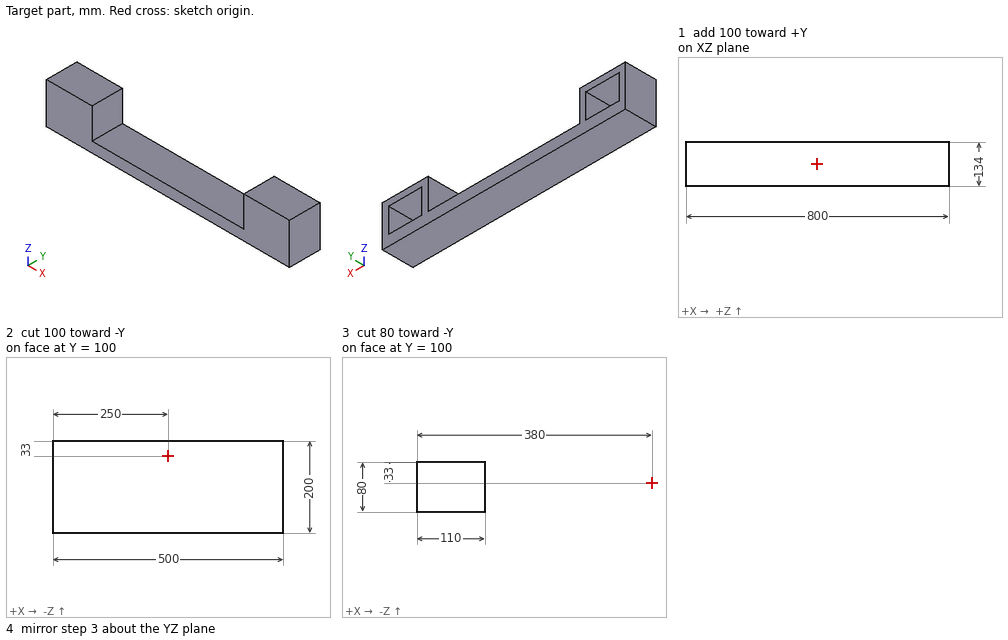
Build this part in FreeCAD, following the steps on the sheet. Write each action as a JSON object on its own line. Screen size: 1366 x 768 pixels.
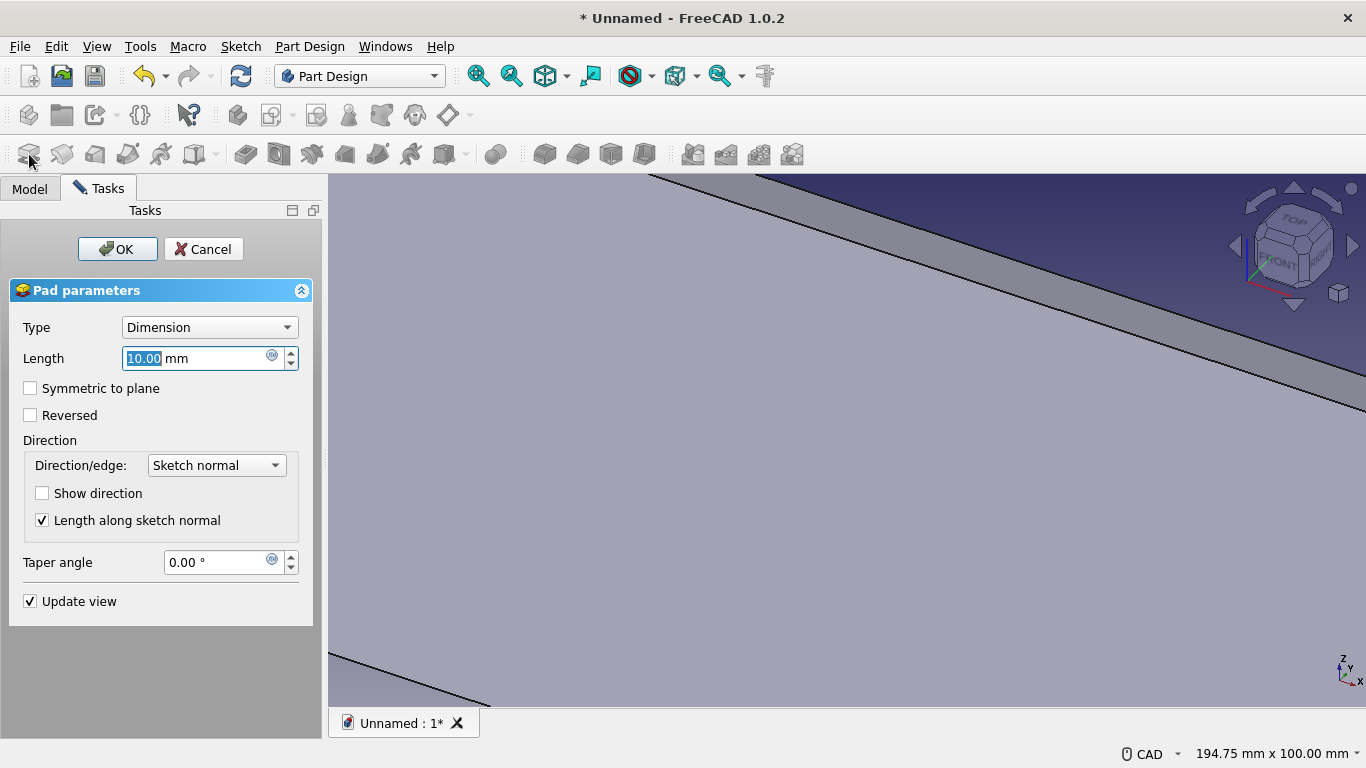
{"action": "type", "text": "100"}
{"action": "key", "text": "Tab"}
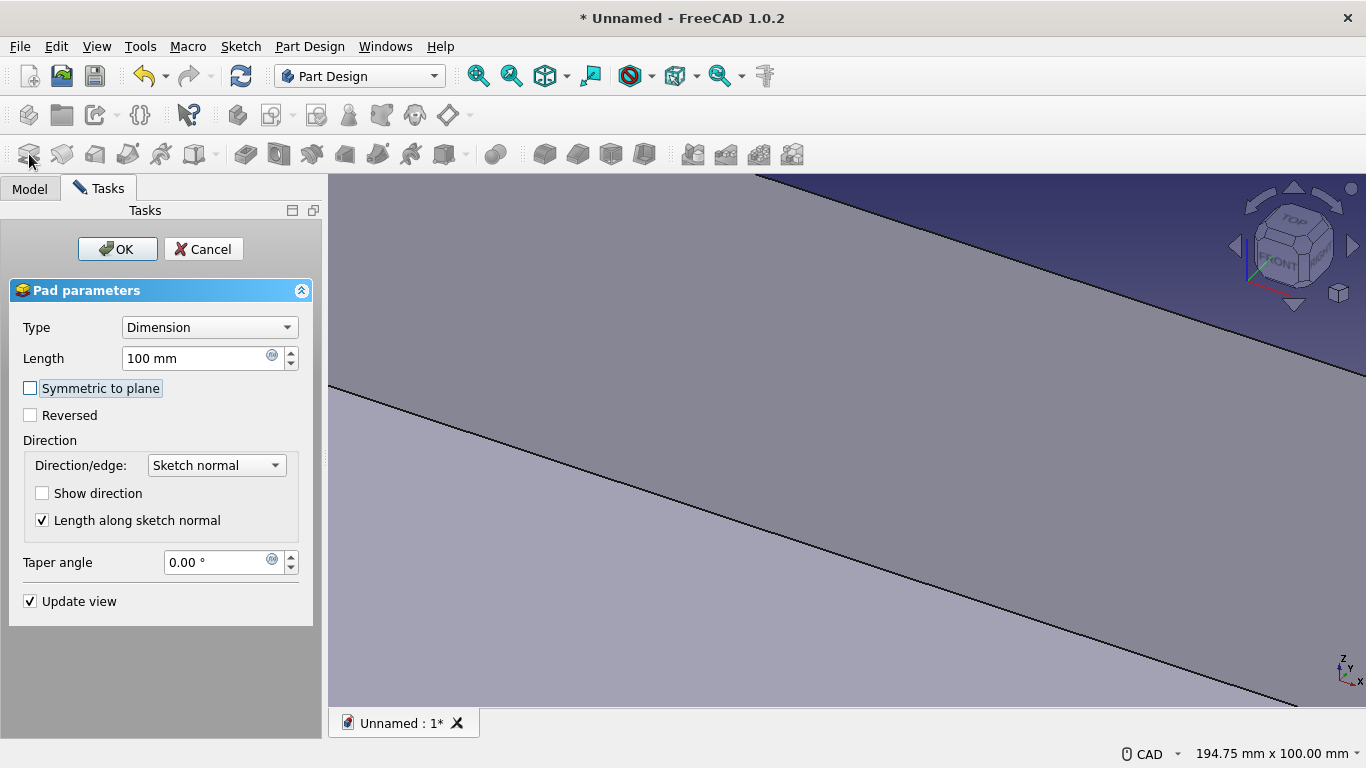
{"action": "left_click", "coordinate": [31, 415]}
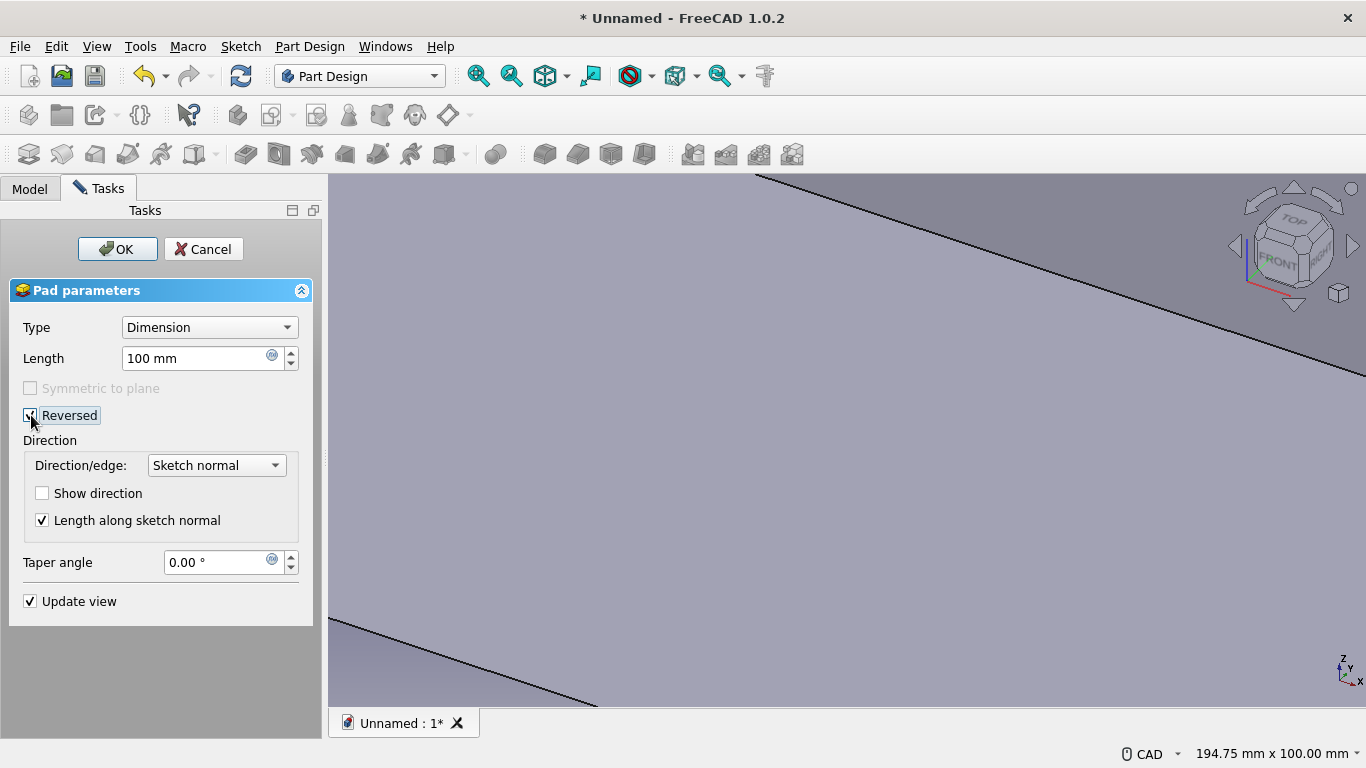
{"action": "left_click", "coordinate": [118, 249]}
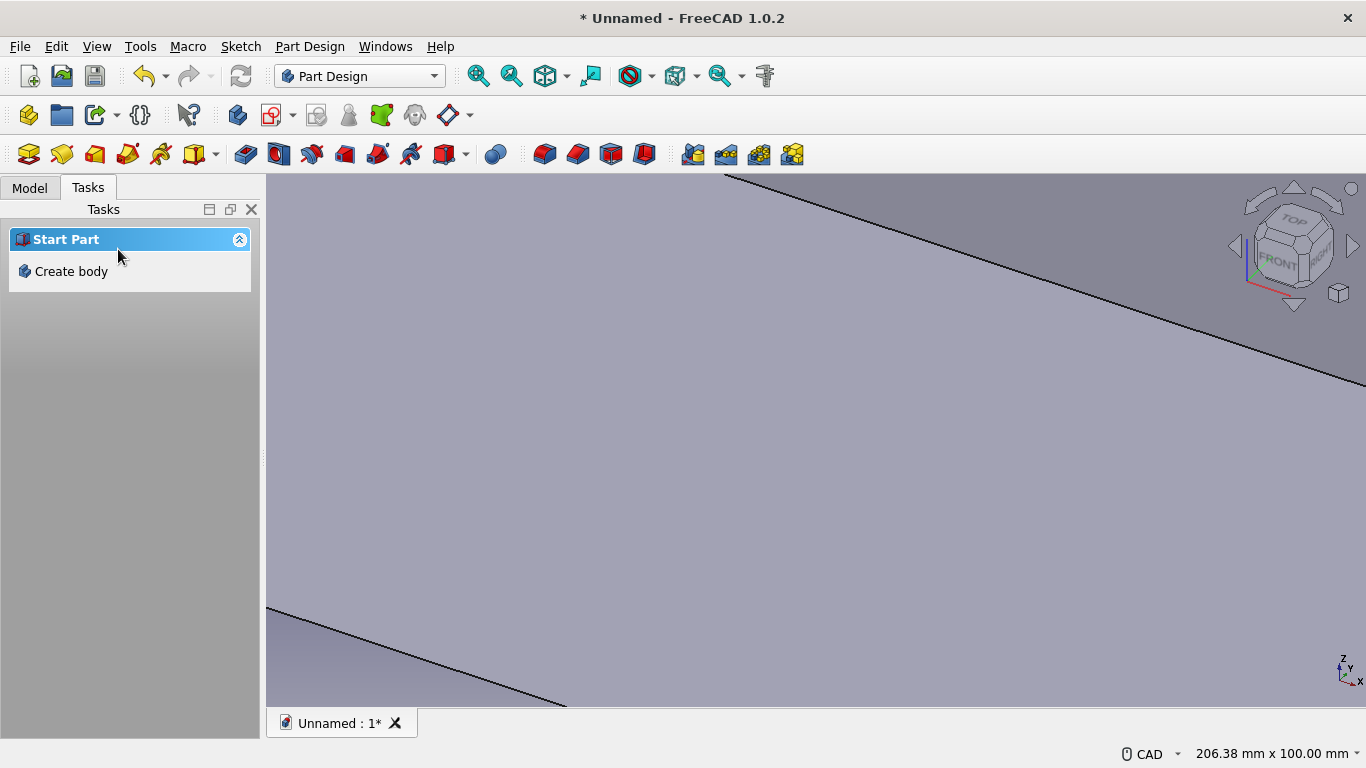
{"action": "key", "text": "v f"}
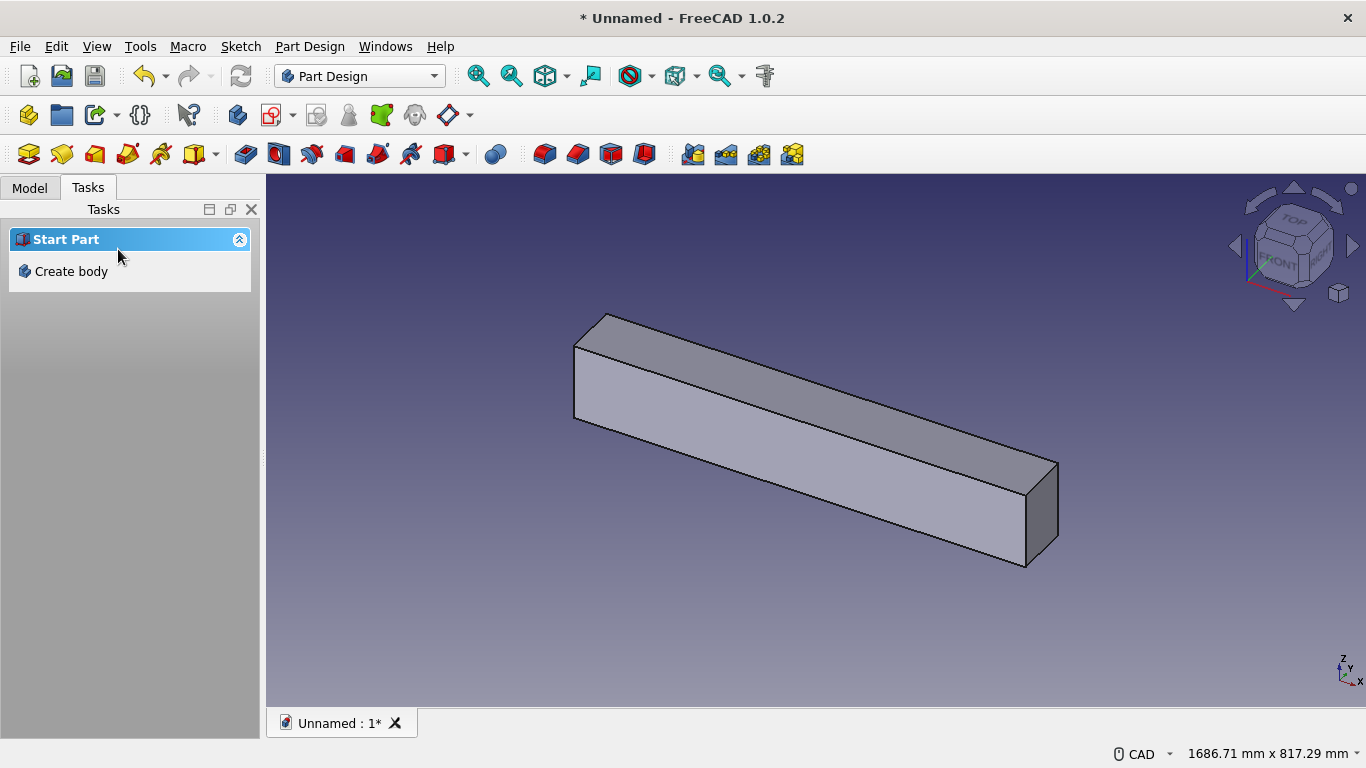
{"action": "key", "text": "4"}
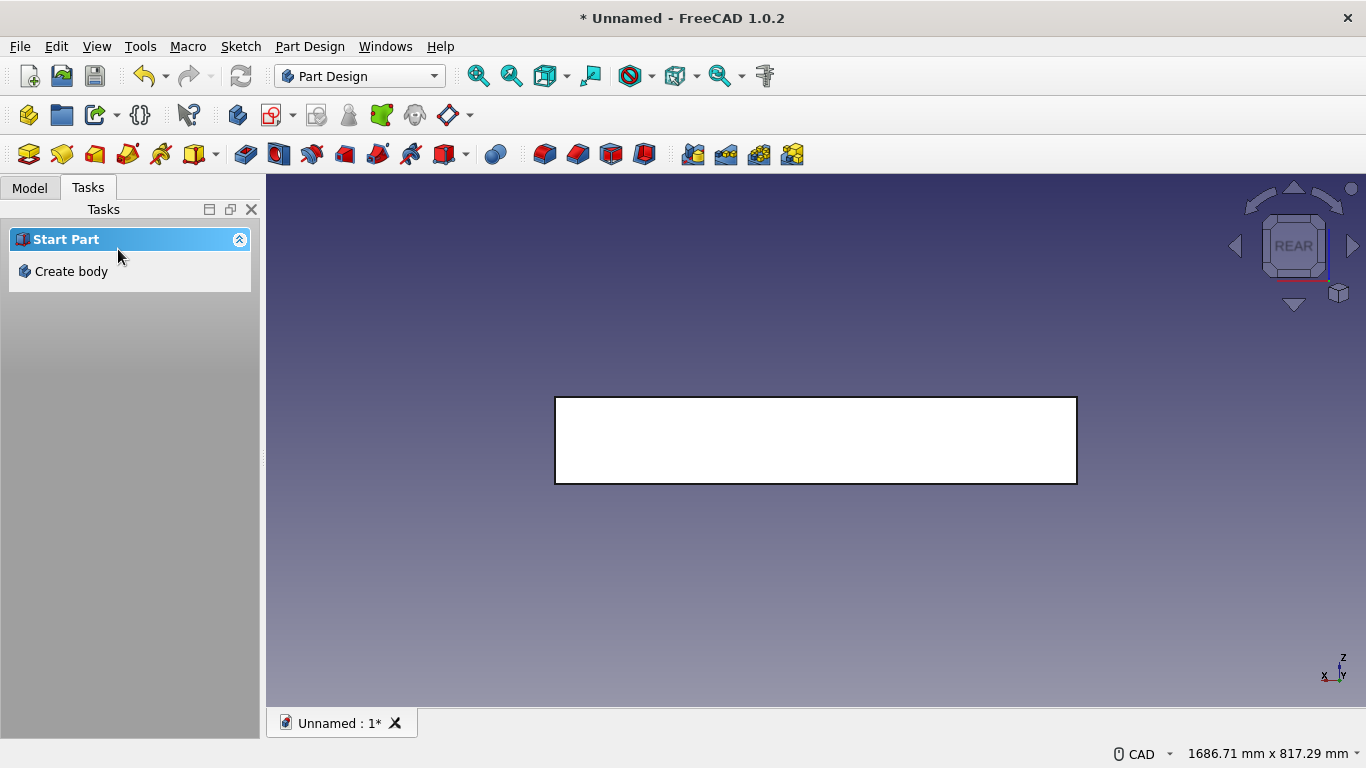
{"action": "left_click", "coordinate": [667, 439]}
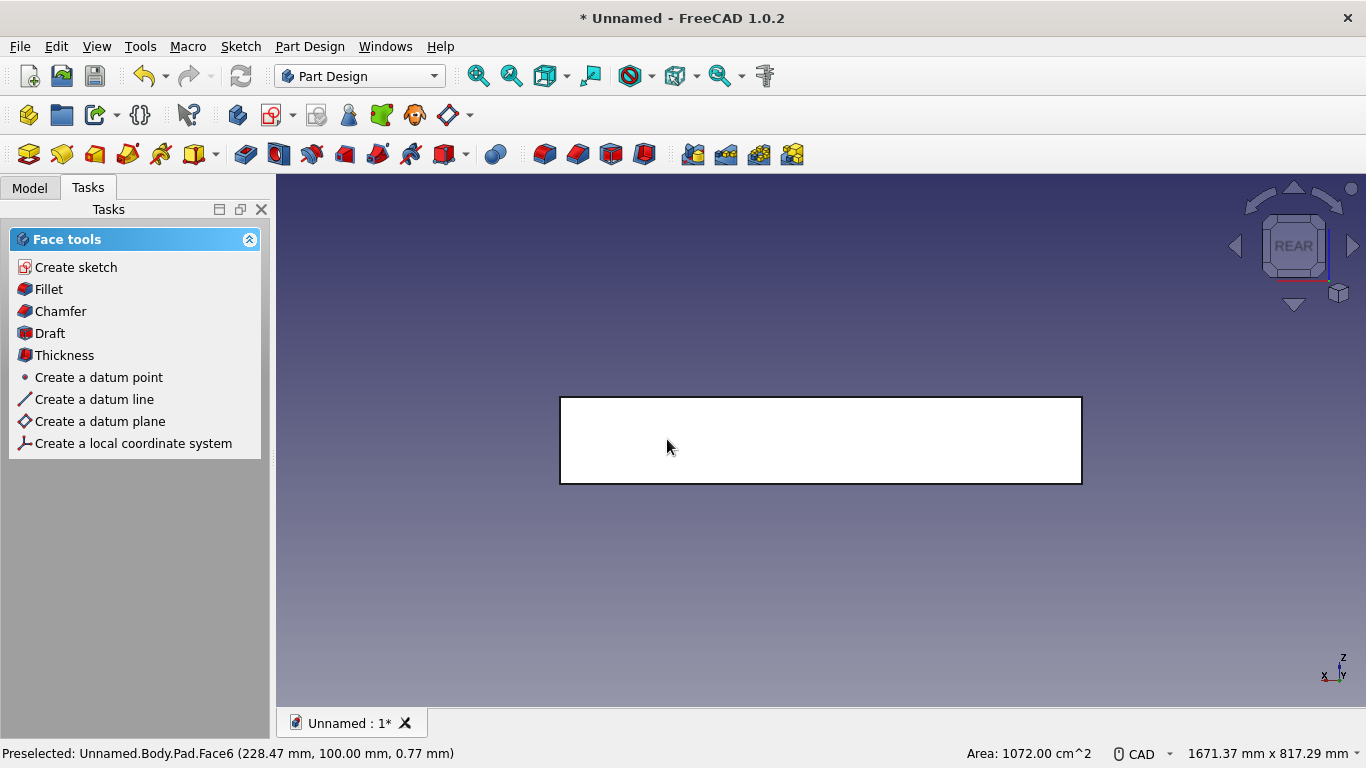
{"action": "left_click", "coordinate": [270, 116]}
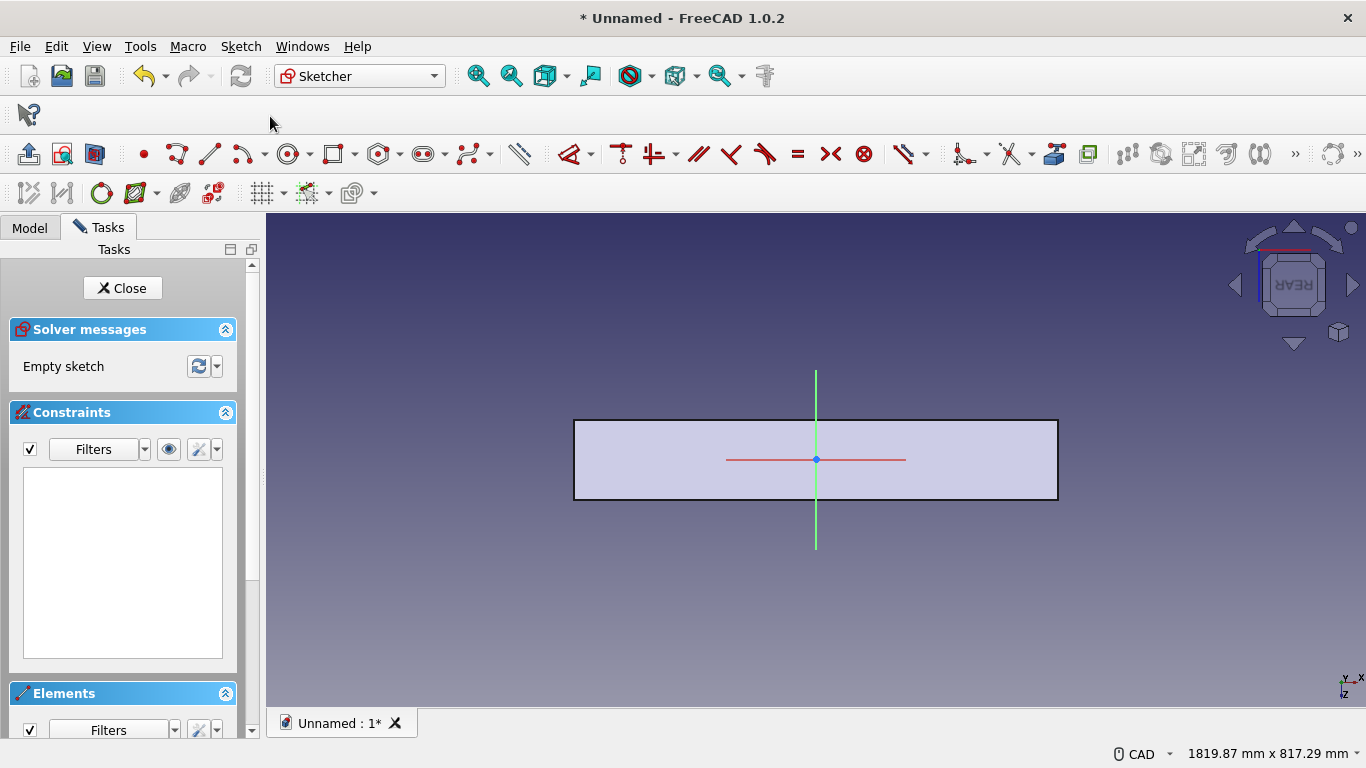
{"action": "scroll", "coordinate": [872, 534], "scroll_direction": "up", "scroll_amount": 4}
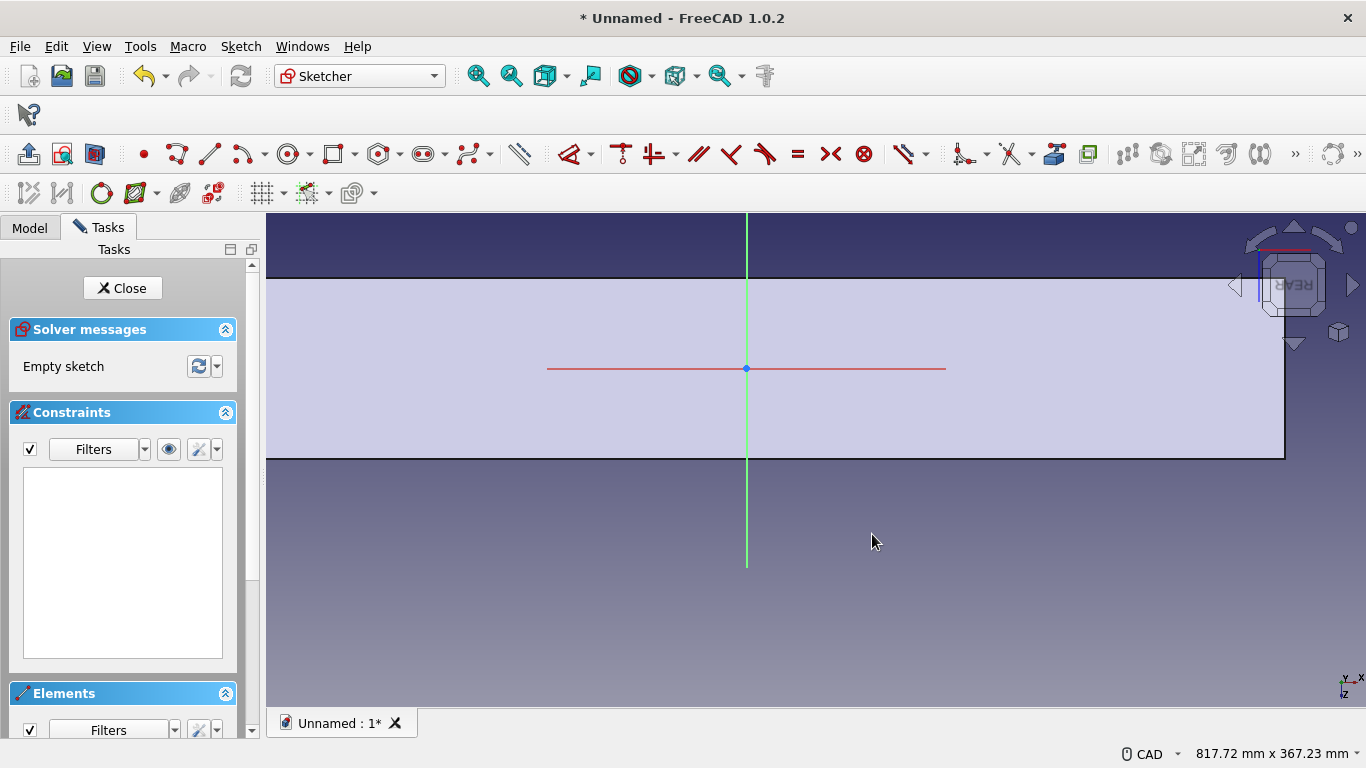
{"action": "left_click", "coordinate": [332, 154]}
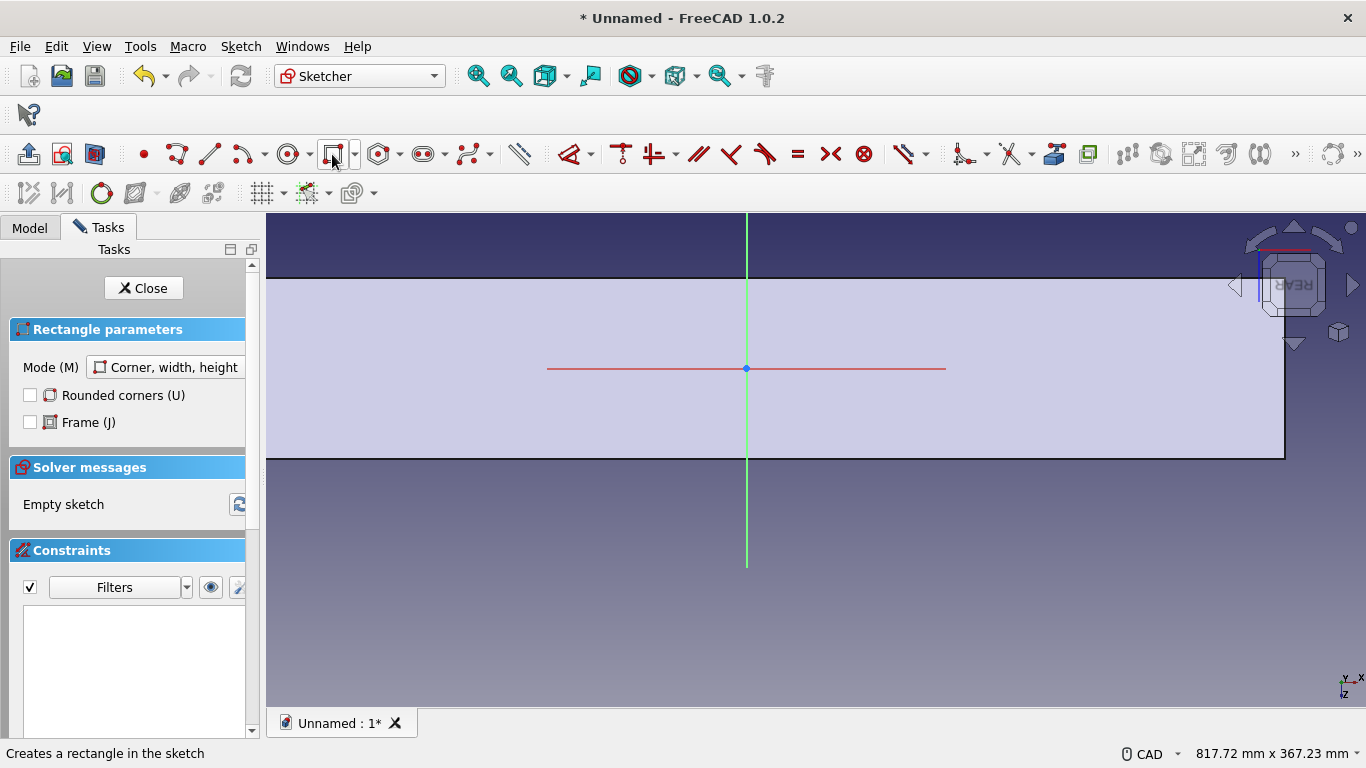
{"action": "left_click", "coordinate": [410, 324]}
{"action": "mouse_move", "coordinate": [1083, 593]}